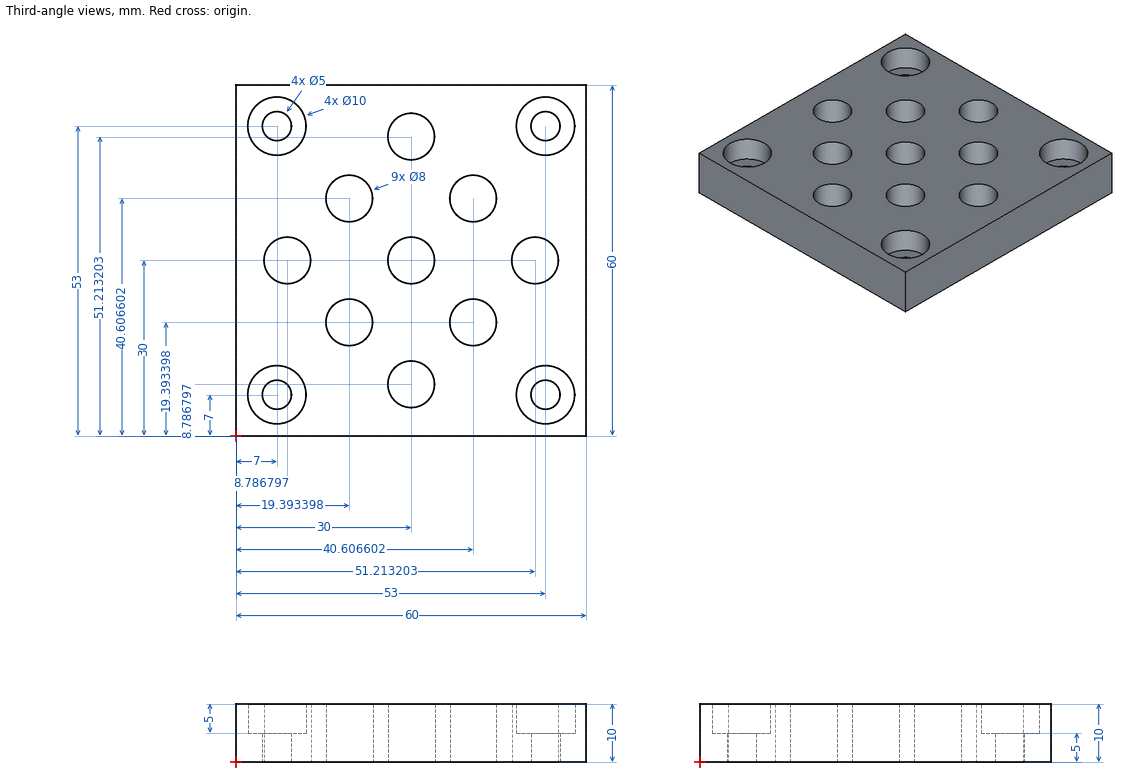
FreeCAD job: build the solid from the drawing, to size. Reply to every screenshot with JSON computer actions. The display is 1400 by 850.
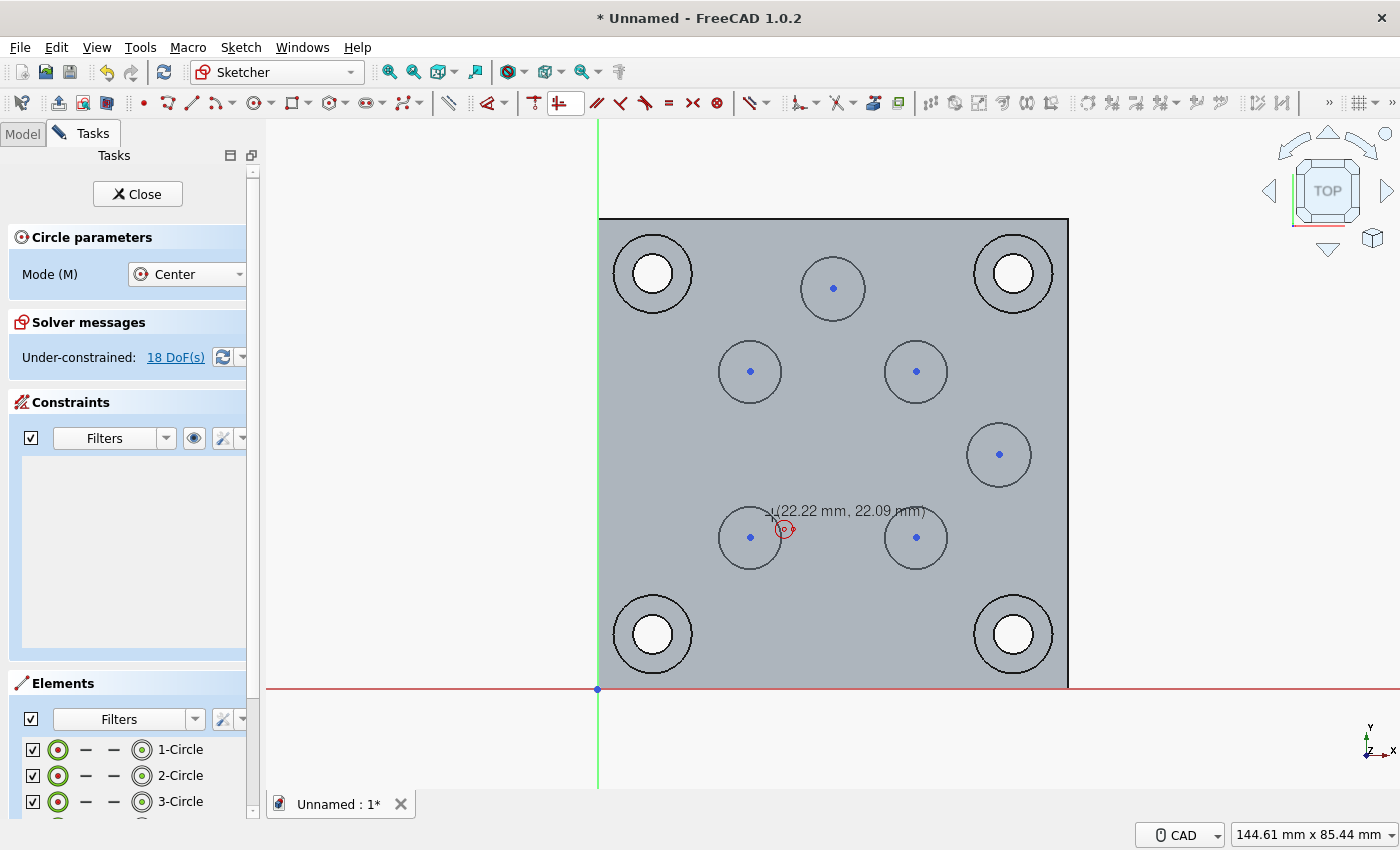
{"action": "left_click", "coordinate": [667, 454]}
{"action": "left_click", "coordinate": [689, 432]}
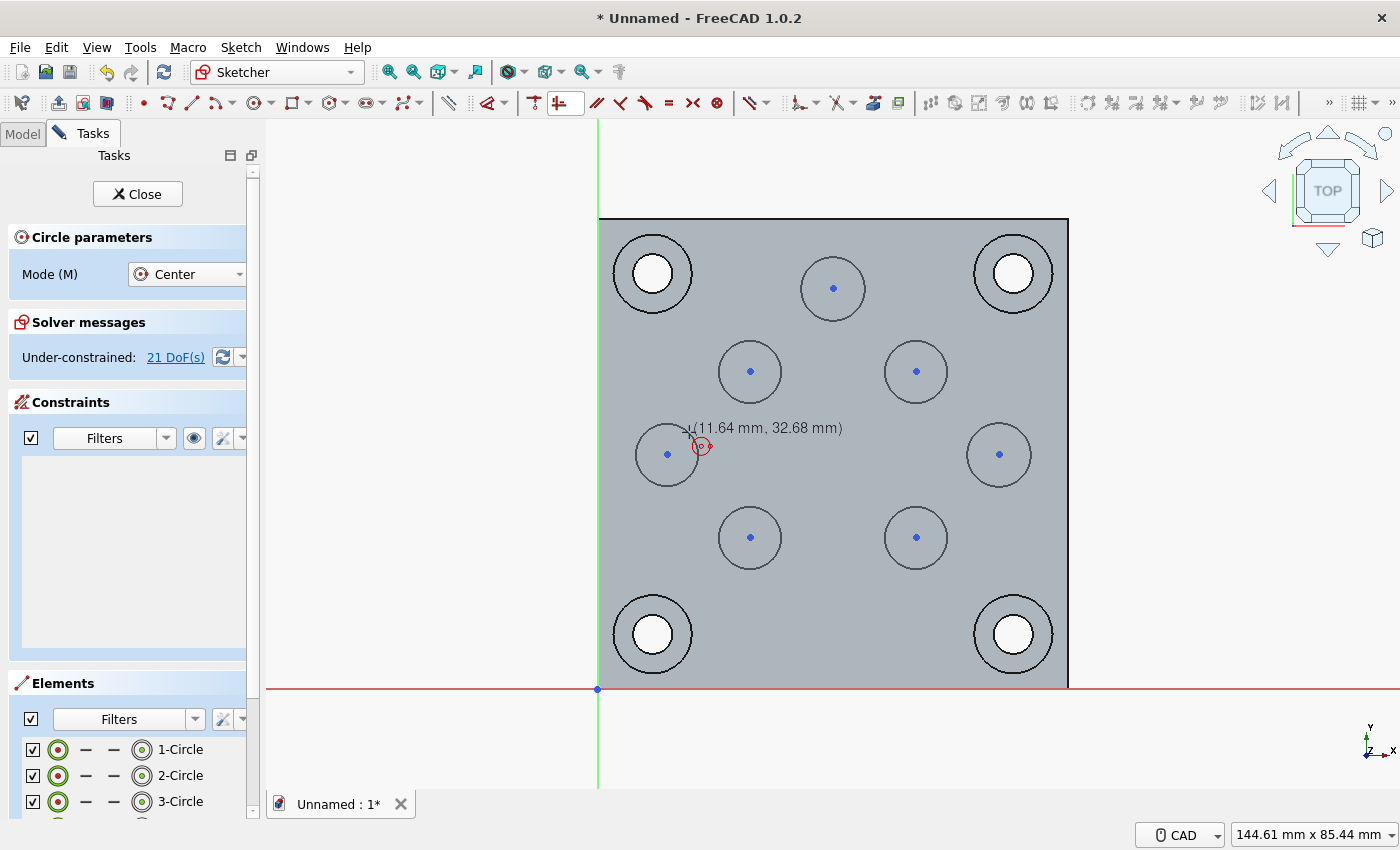
{"action": "left_click", "coordinate": [833, 620]}
{"action": "left_click", "coordinate": [855, 598]}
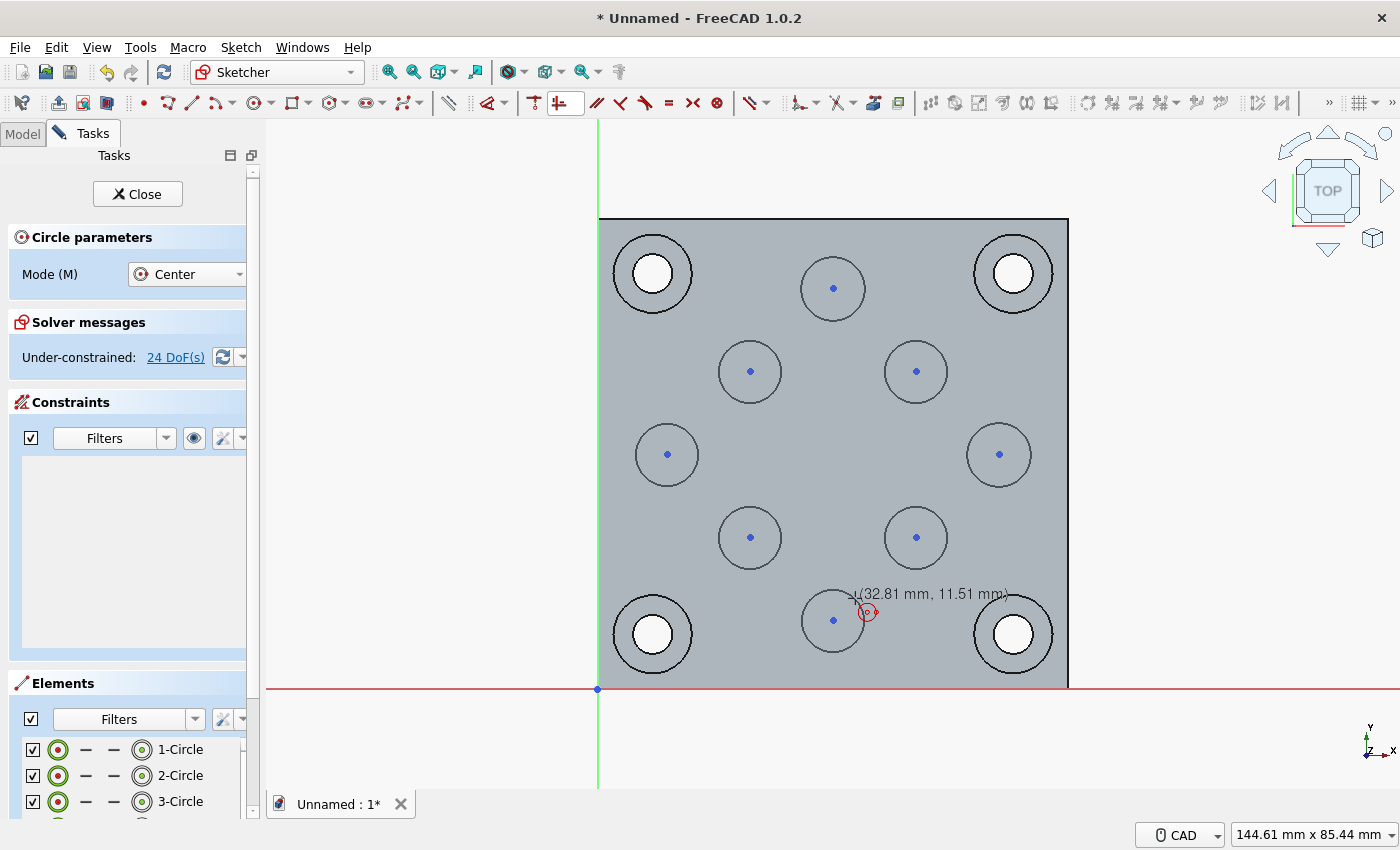
{"action": "left_click", "coordinate": [833, 454]}
{"action": "left_click", "coordinate": [855, 432]}
{"action": "key", "text": "Escape"}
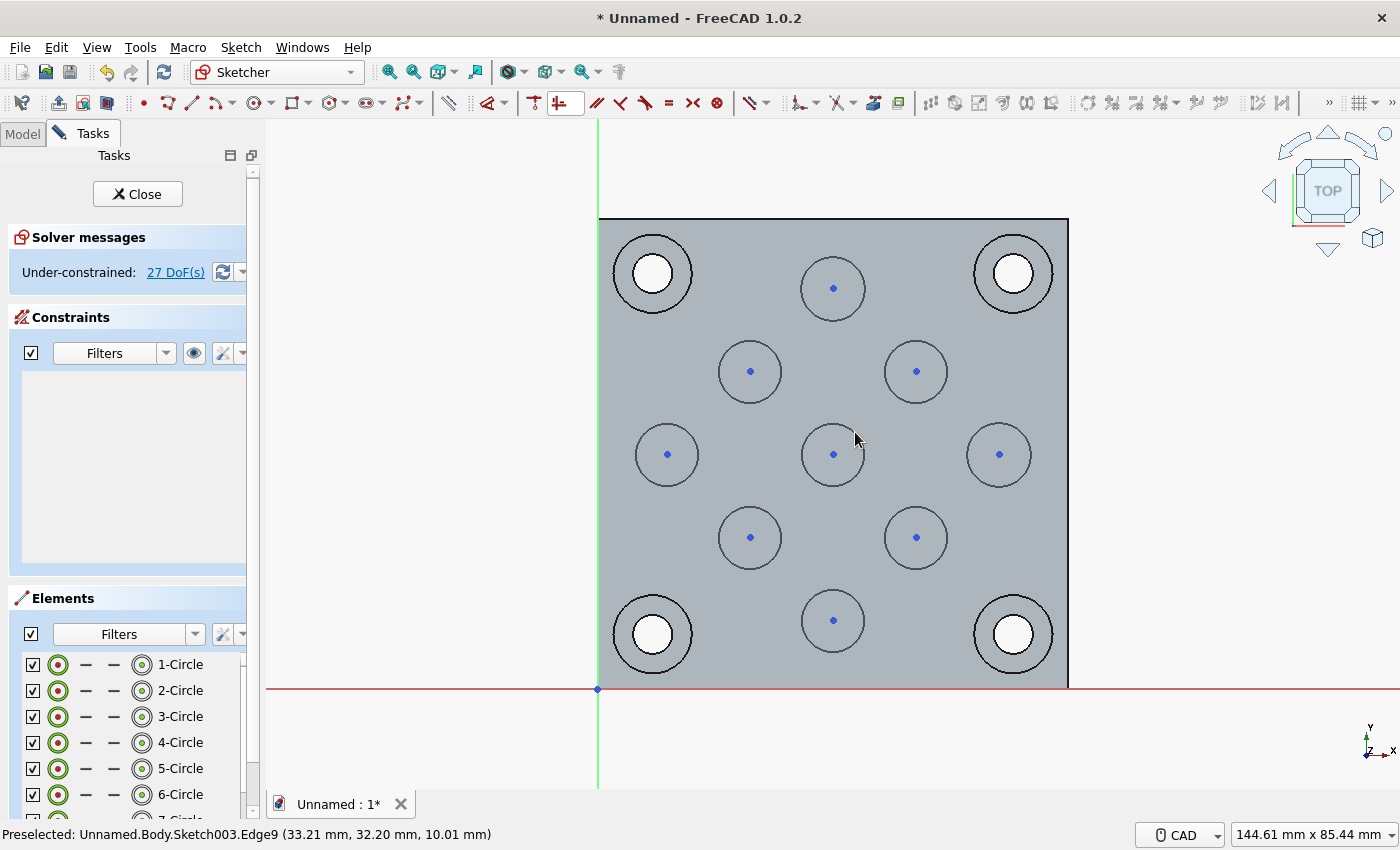
{"action": "left_click", "coordinate": [772, 350]}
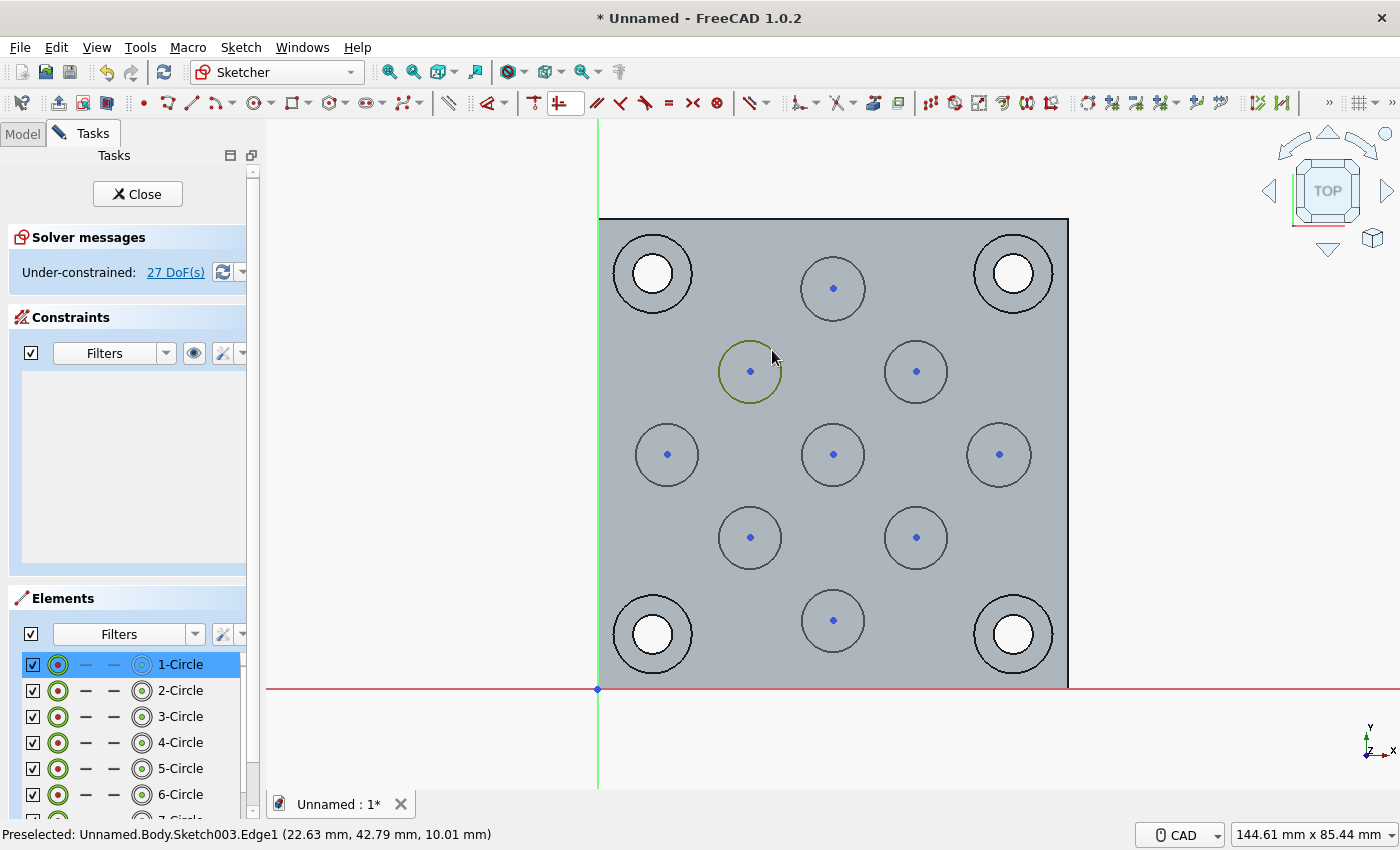
{"action": "left_click", "coordinate": [855, 266]}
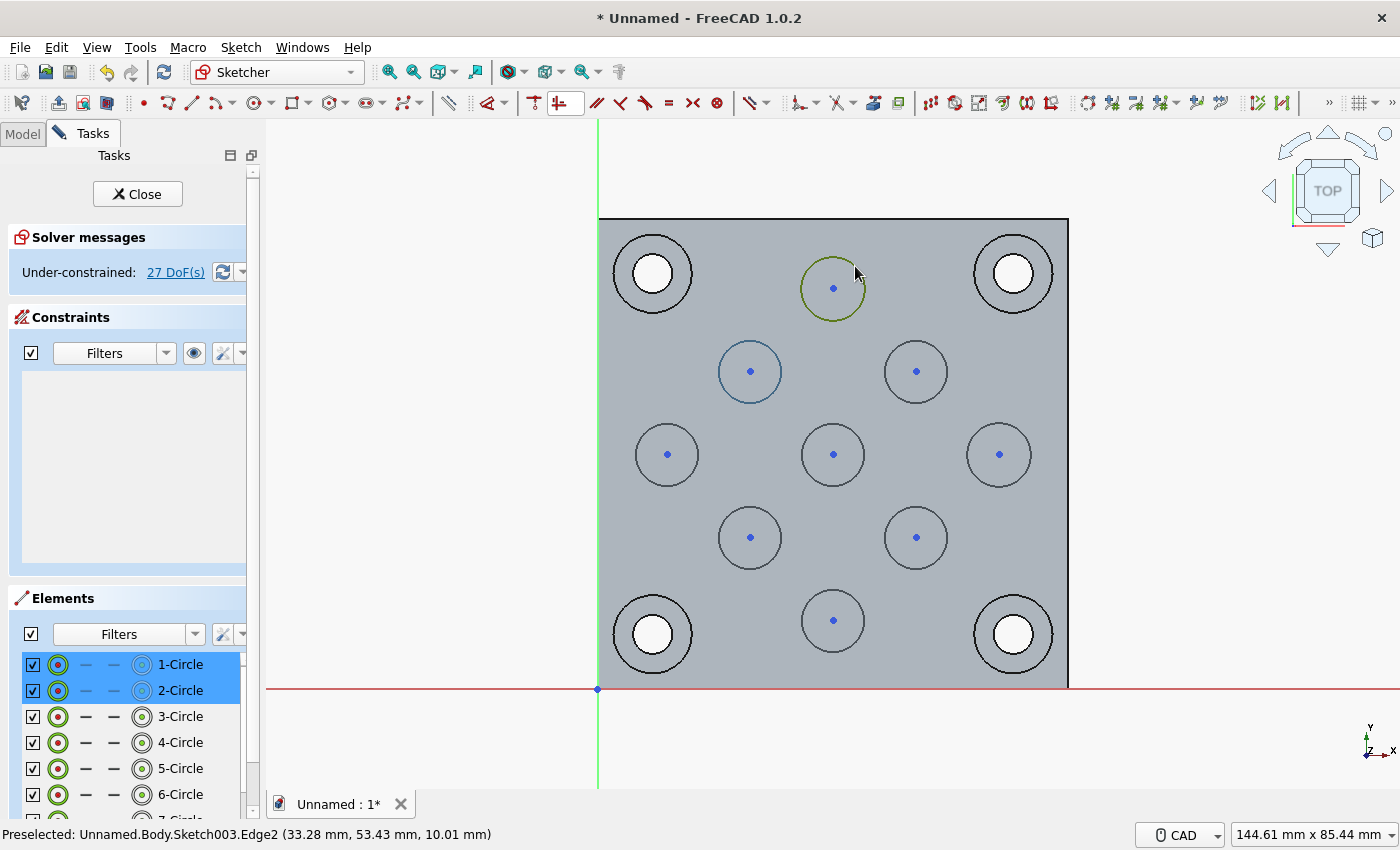
{"action": "left_click", "coordinate": [938, 350]}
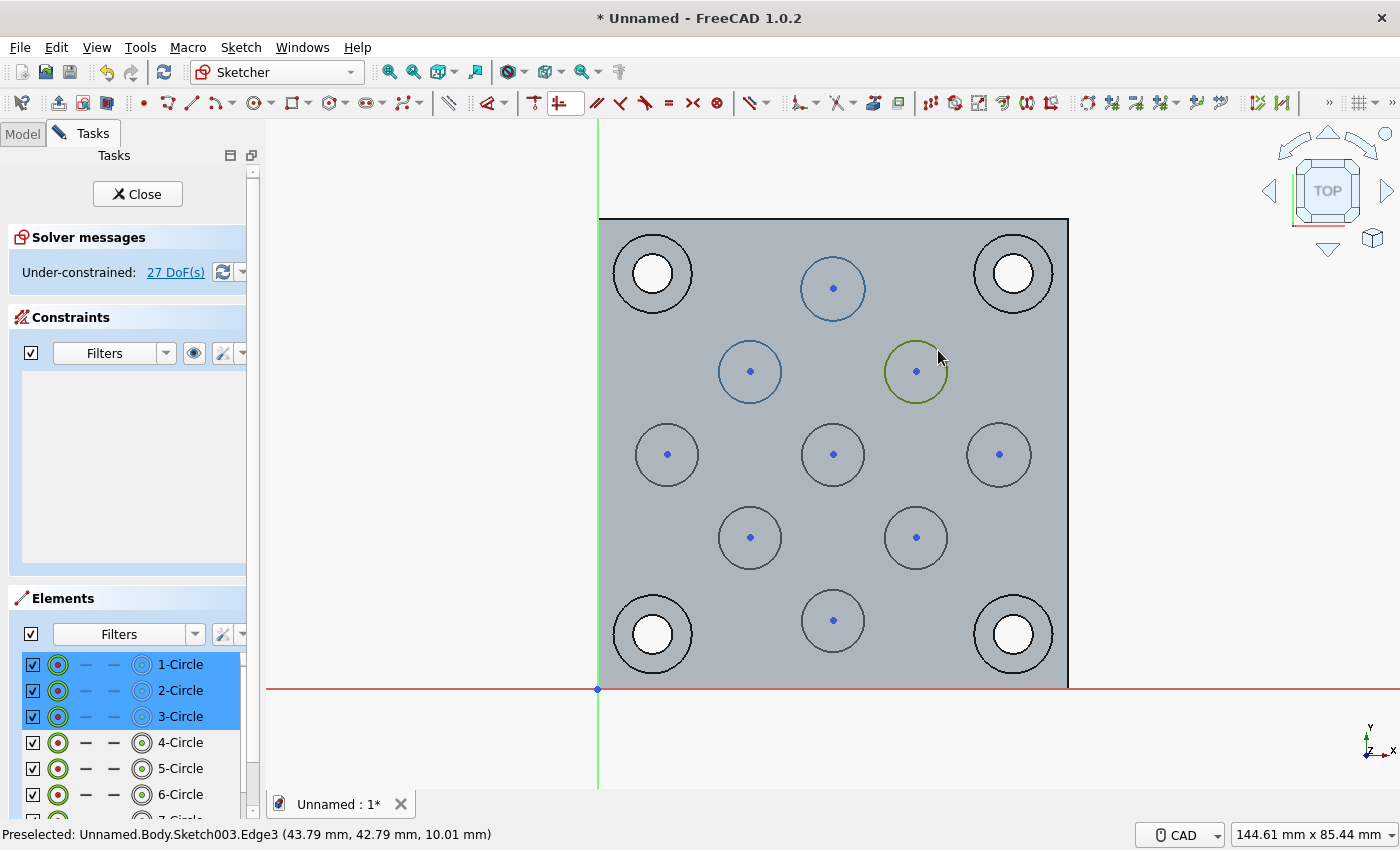
{"action": "left_click", "coordinate": [1021, 432]}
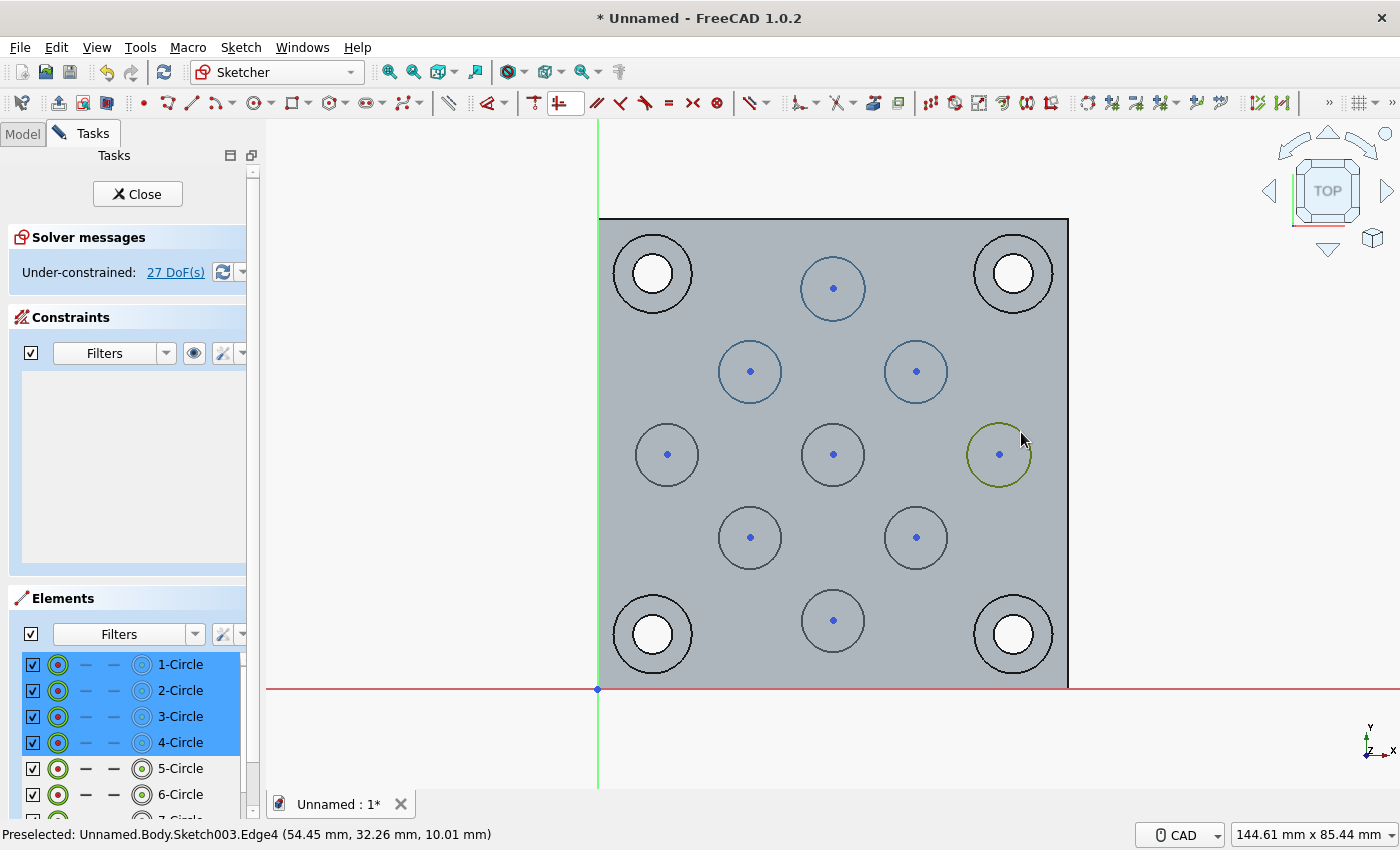
{"action": "left_click", "coordinate": [938, 516]}